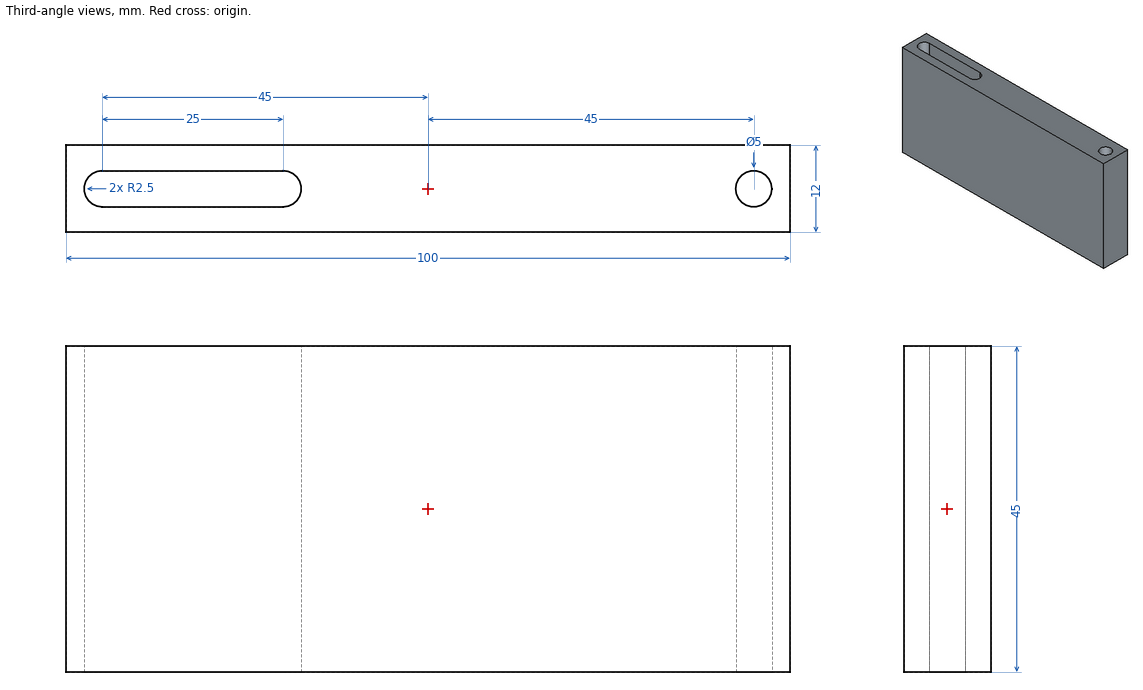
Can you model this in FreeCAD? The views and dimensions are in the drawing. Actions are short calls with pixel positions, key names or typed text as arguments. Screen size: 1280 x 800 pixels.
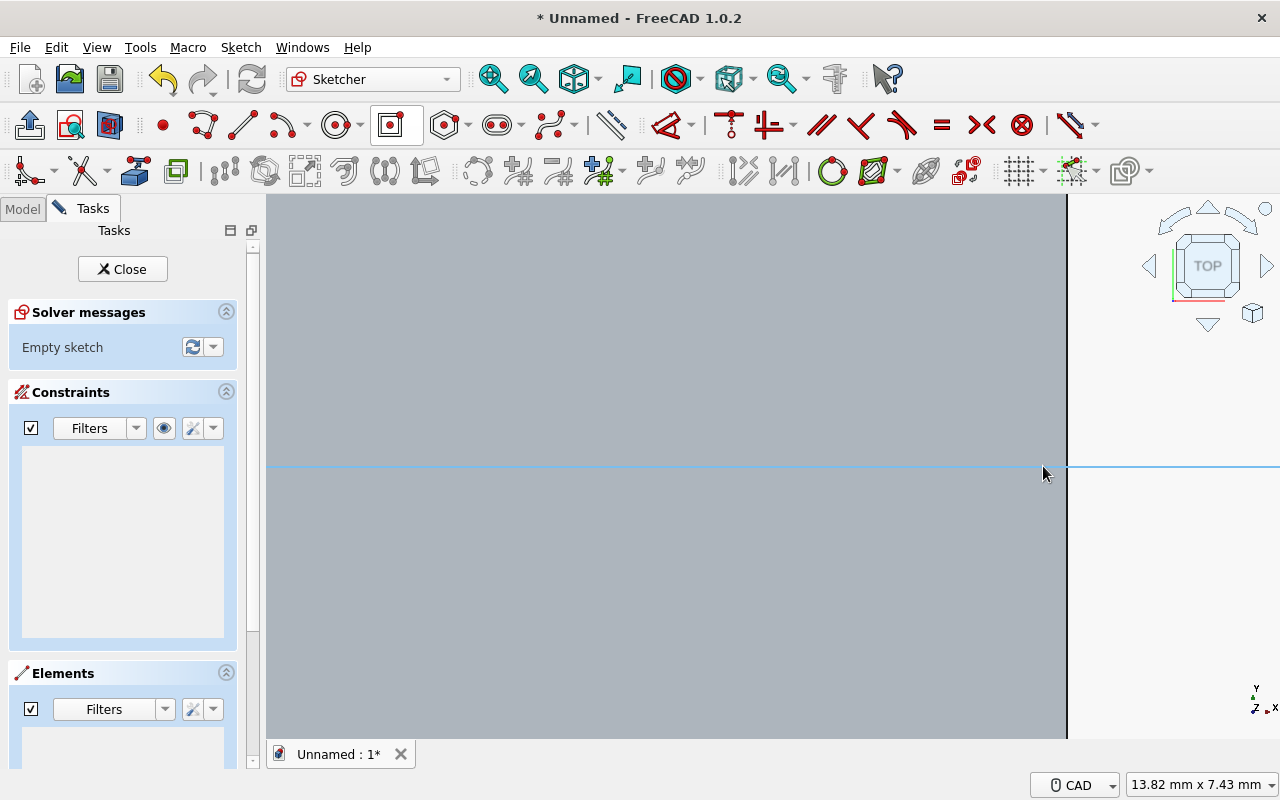
click(336, 126)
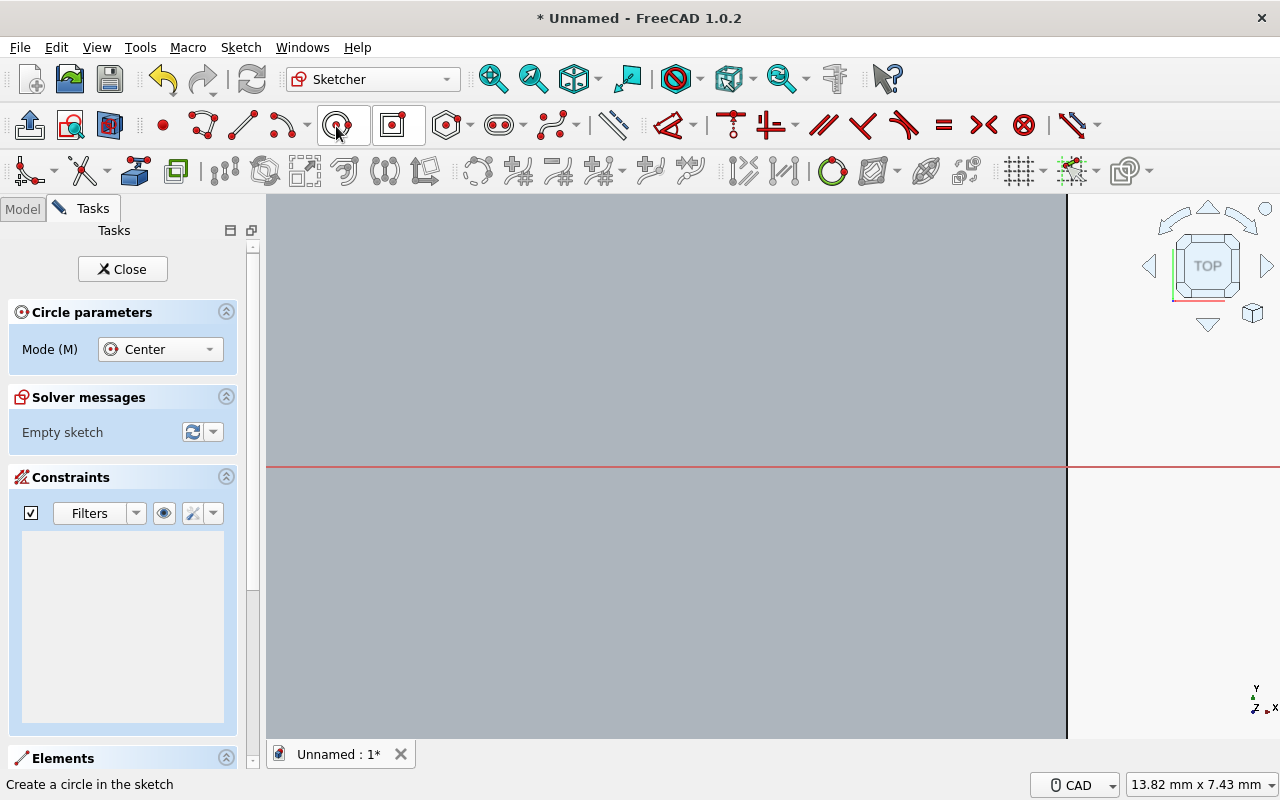
click(700, 466)
click(830, 337)
key(Escape)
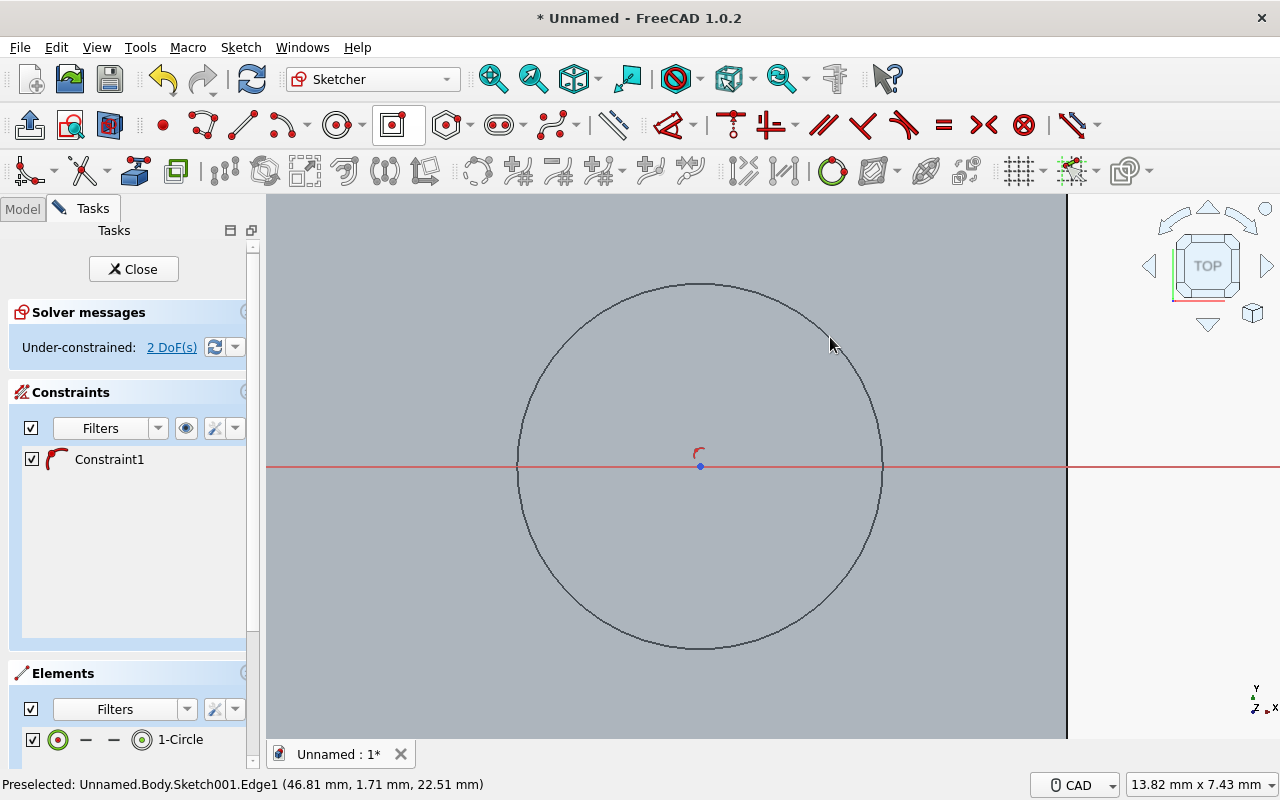
click(668, 126)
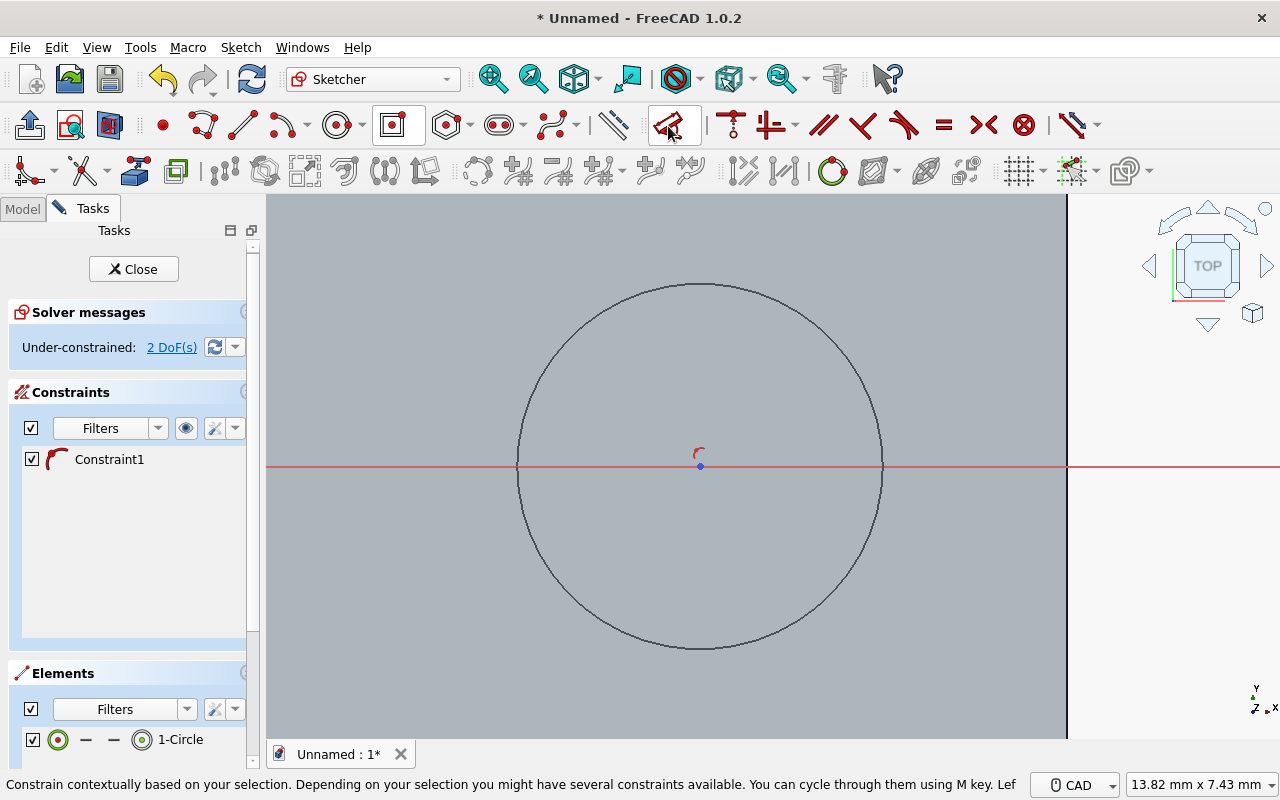
click(829, 337)
click(852, 314)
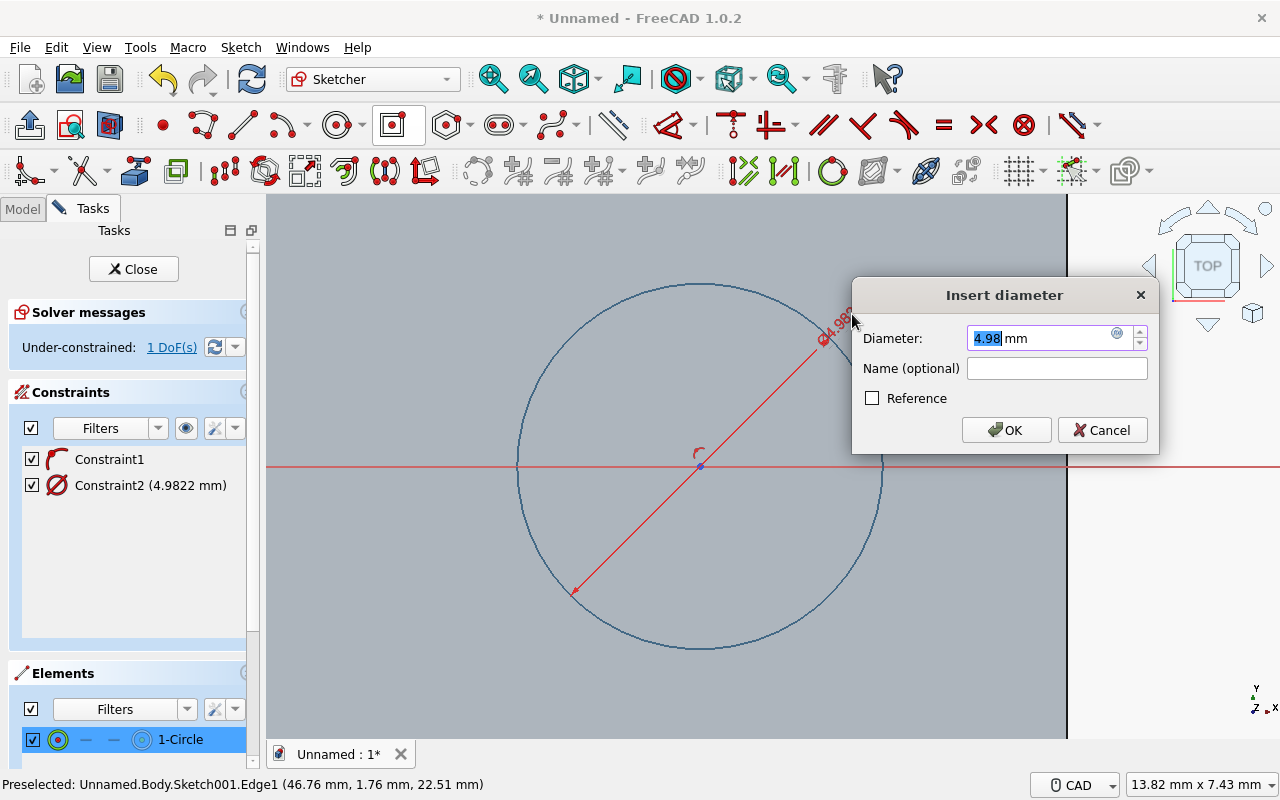
text(5)
key(Return)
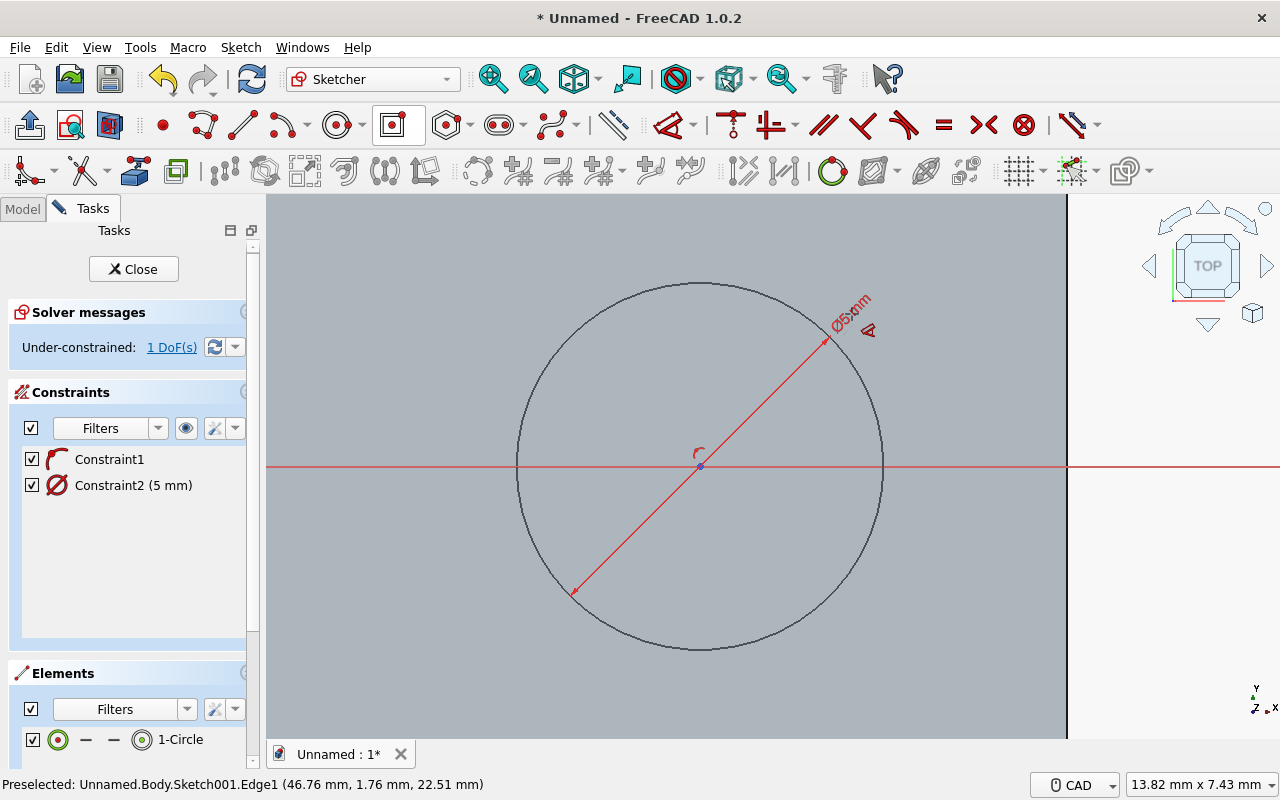
click(700, 466)
click(497, 500)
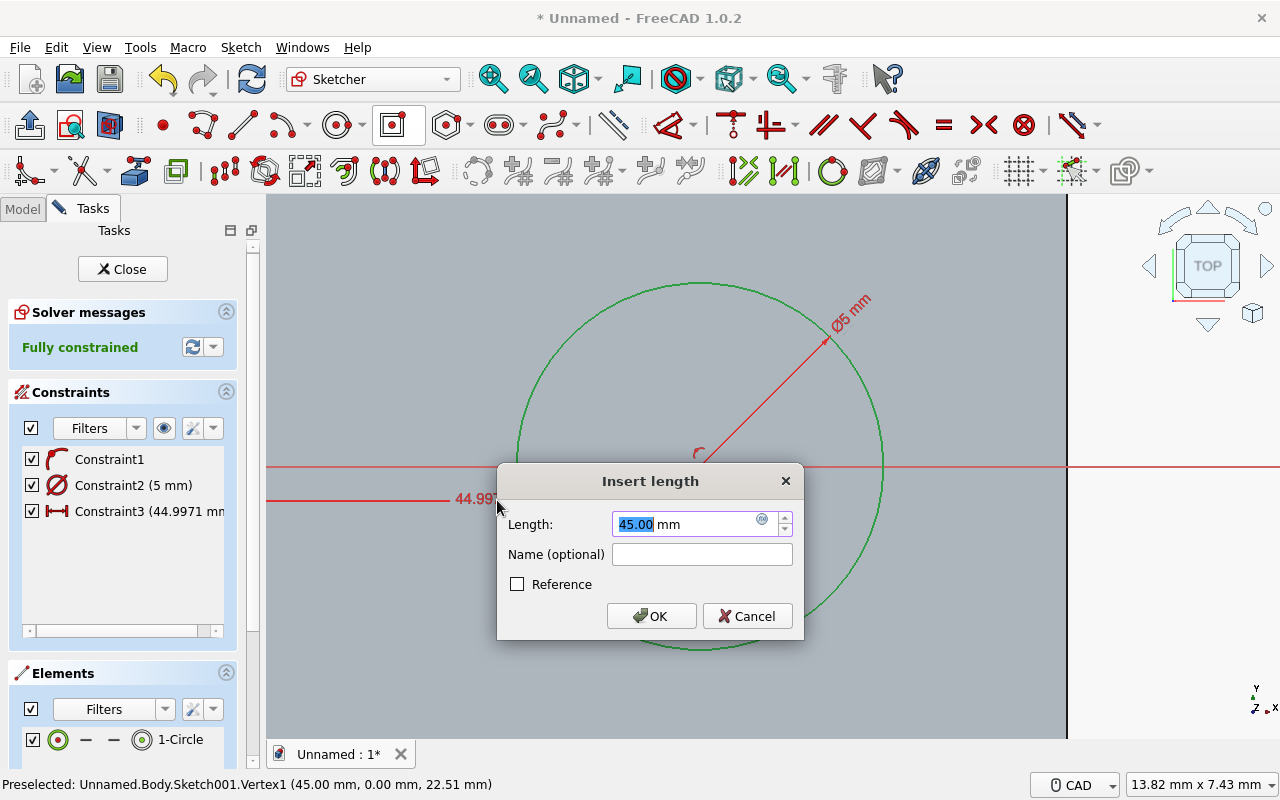
text(45)
key(Return)
key(Escape)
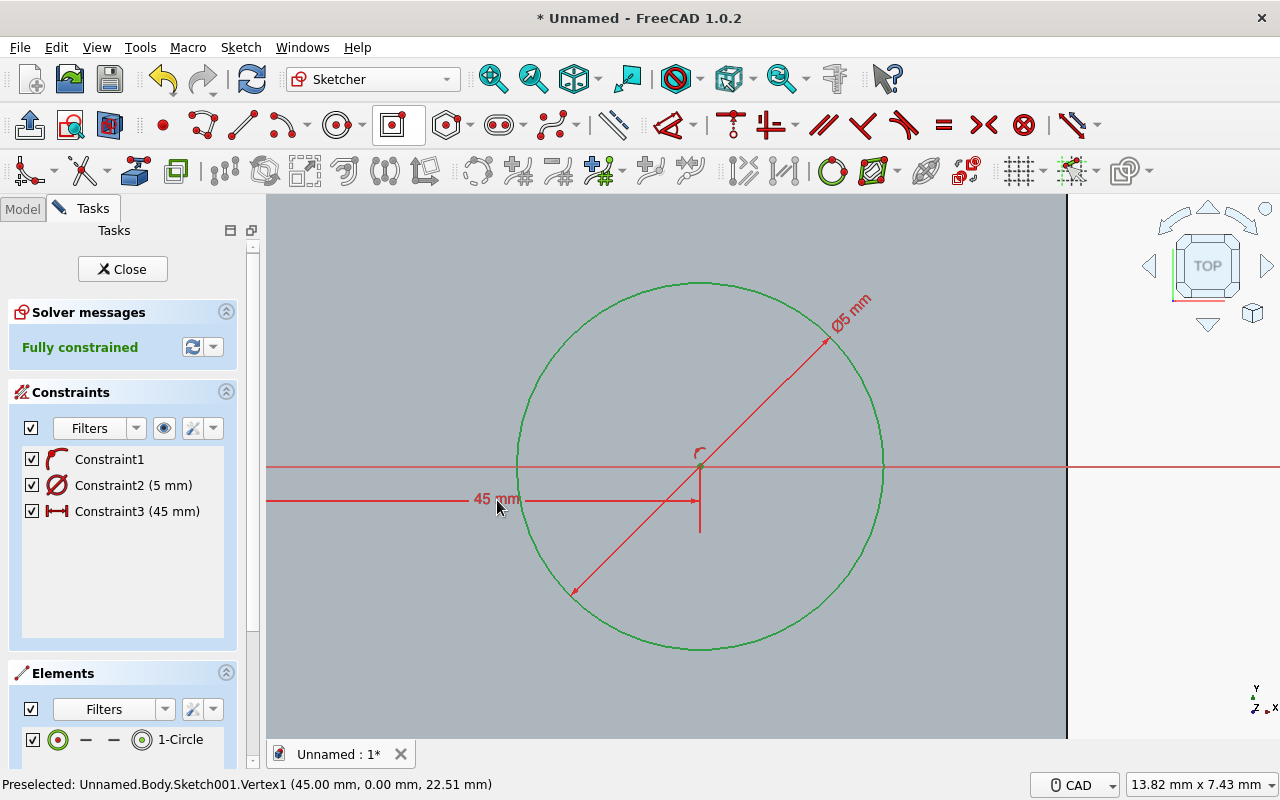
click(123, 269)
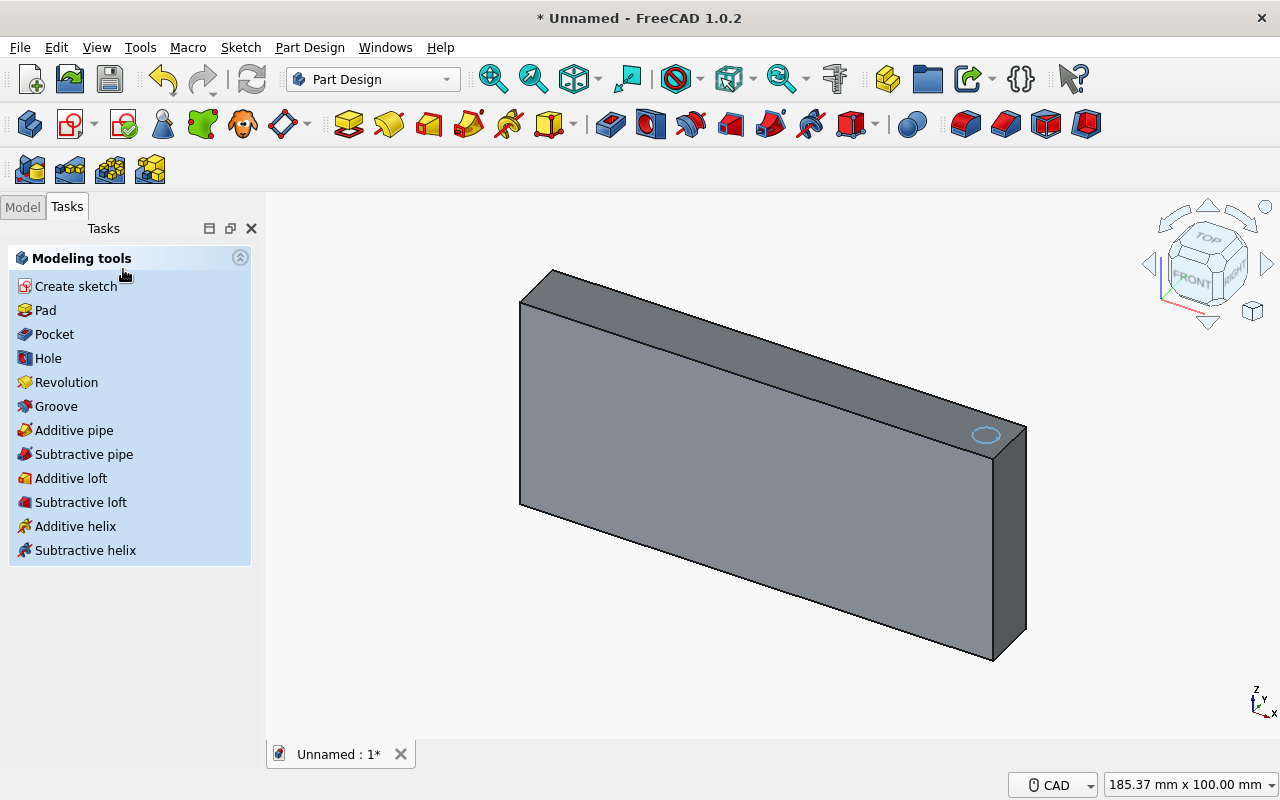
click(612, 124)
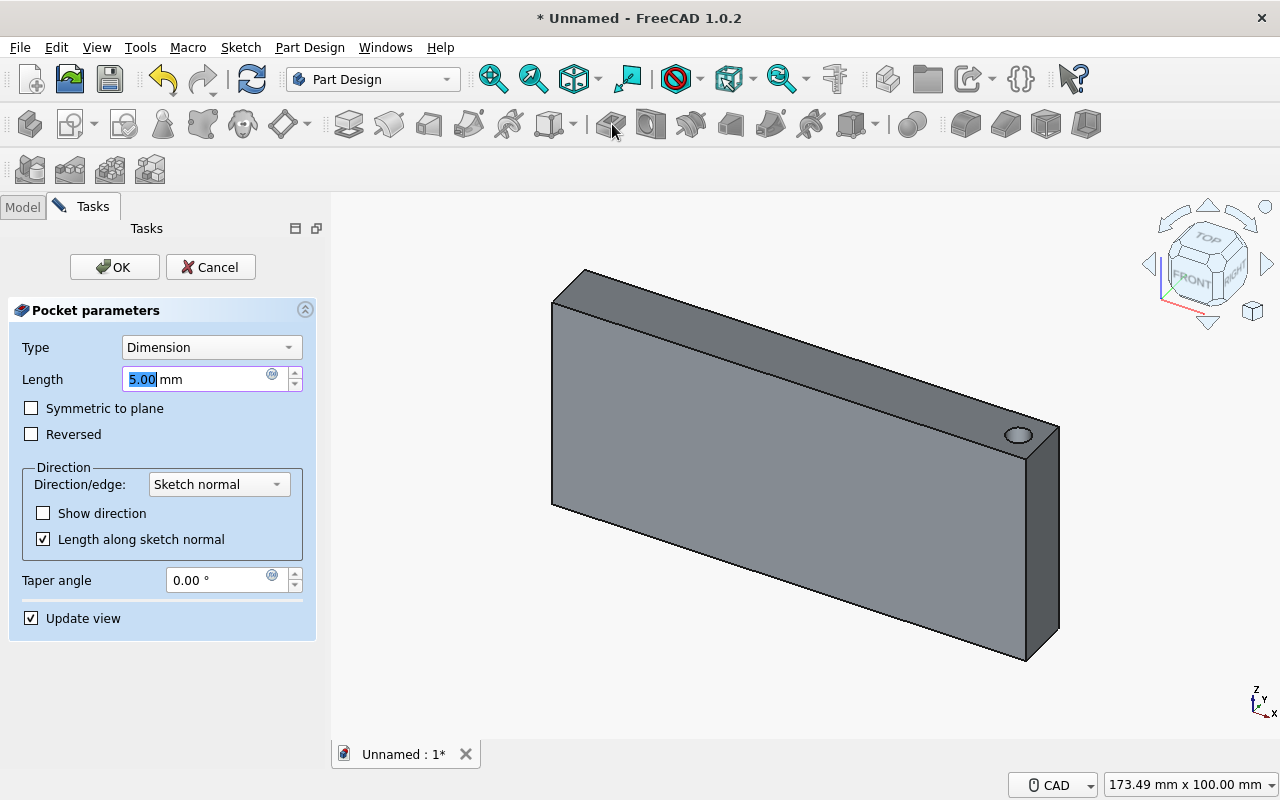
click(212, 348)